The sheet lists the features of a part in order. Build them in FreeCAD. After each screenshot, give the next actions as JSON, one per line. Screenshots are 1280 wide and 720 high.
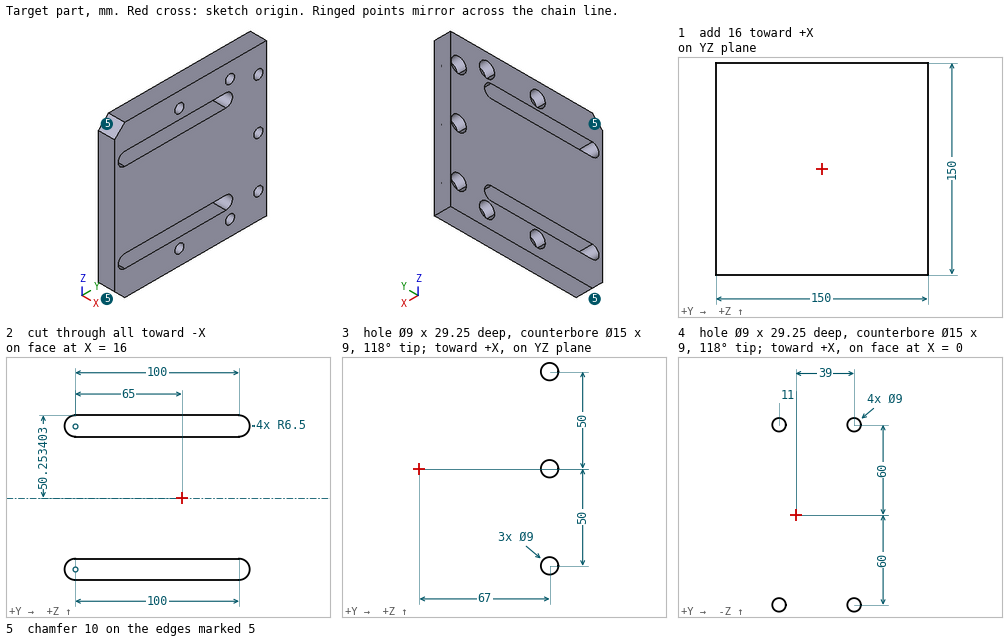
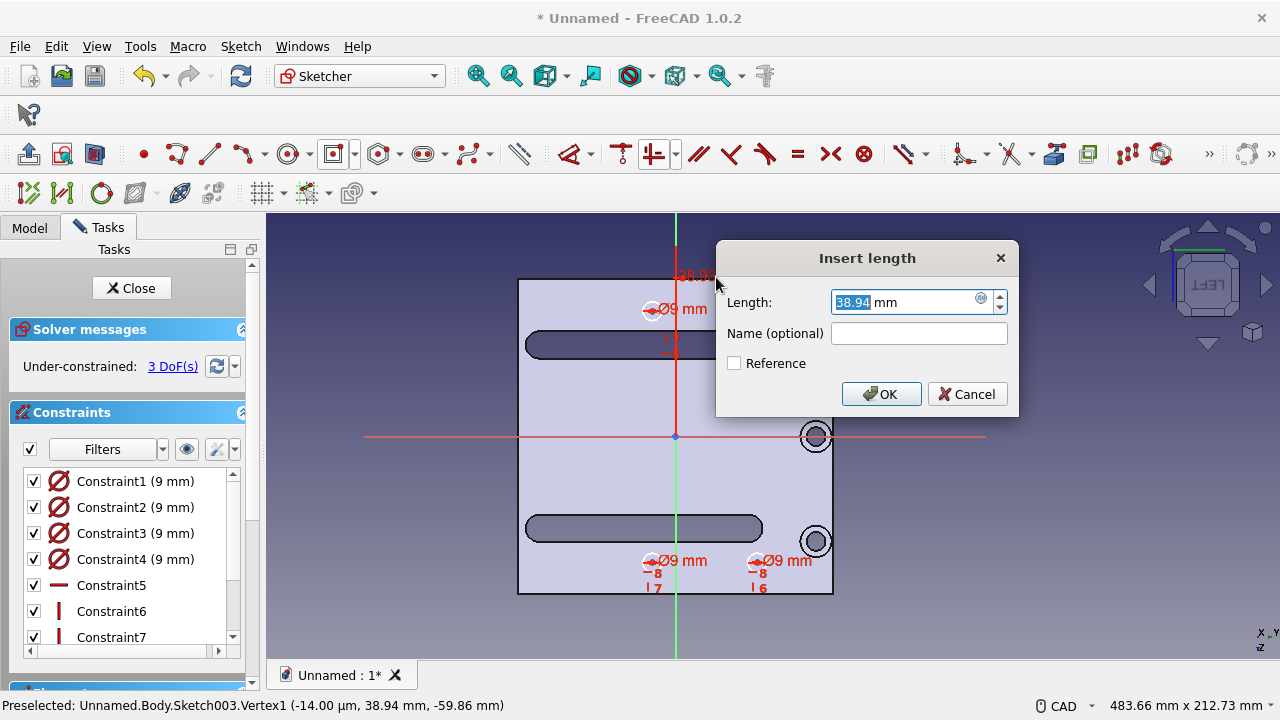
{"action": "type", "text": "39"}
{"action": "key", "text": "Return"}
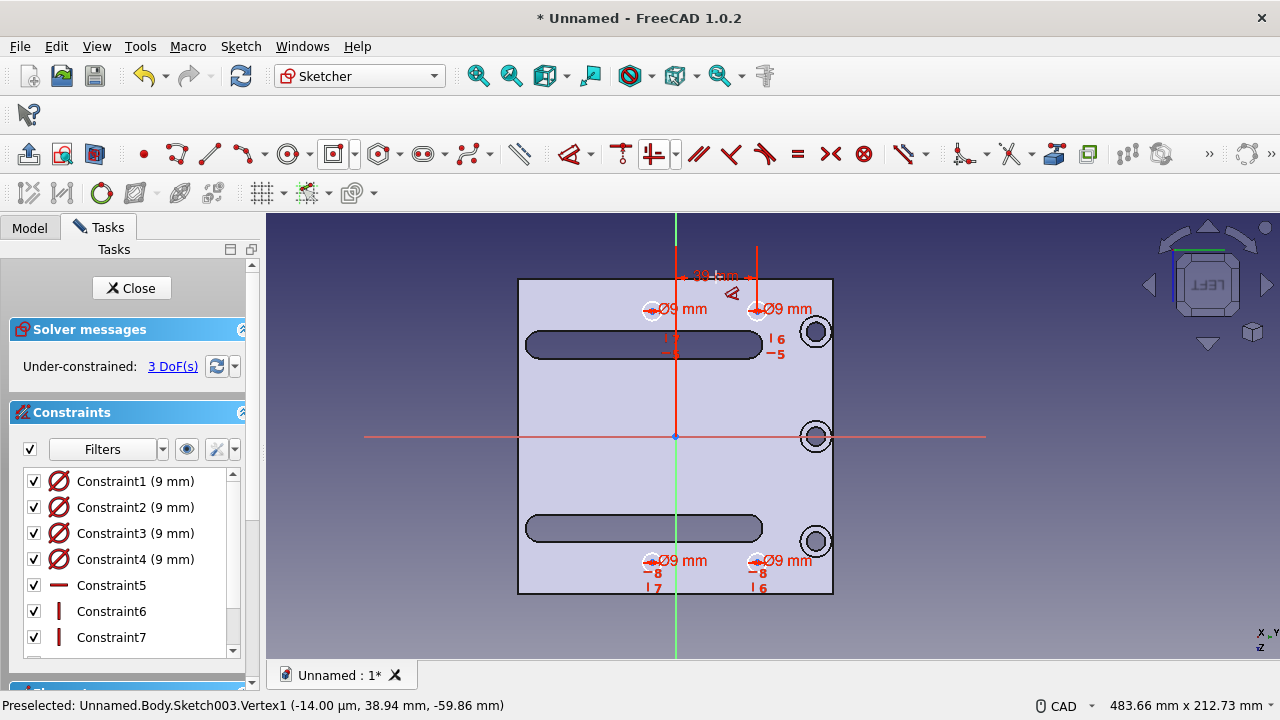
{"action": "left_click", "coordinate": [757, 311]}
{"action": "left_click", "coordinate": [791, 374]}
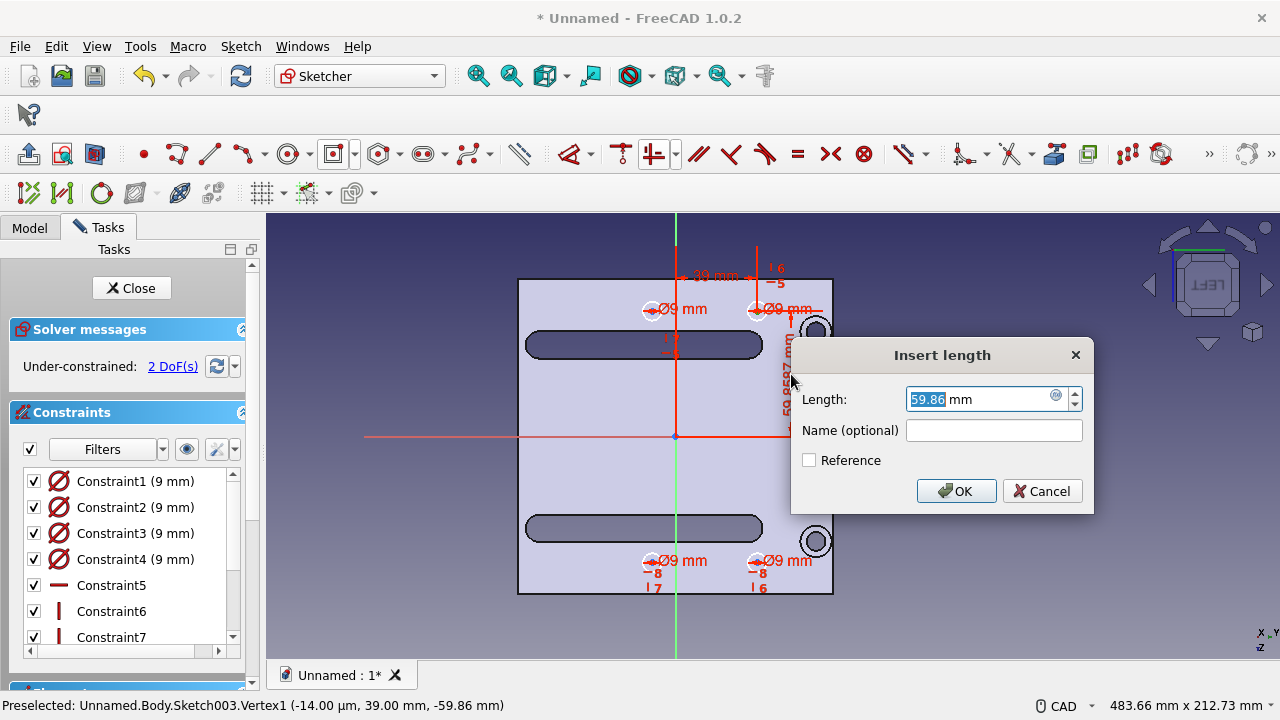
{"action": "type", "text": "60"}
{"action": "key", "text": "Return"}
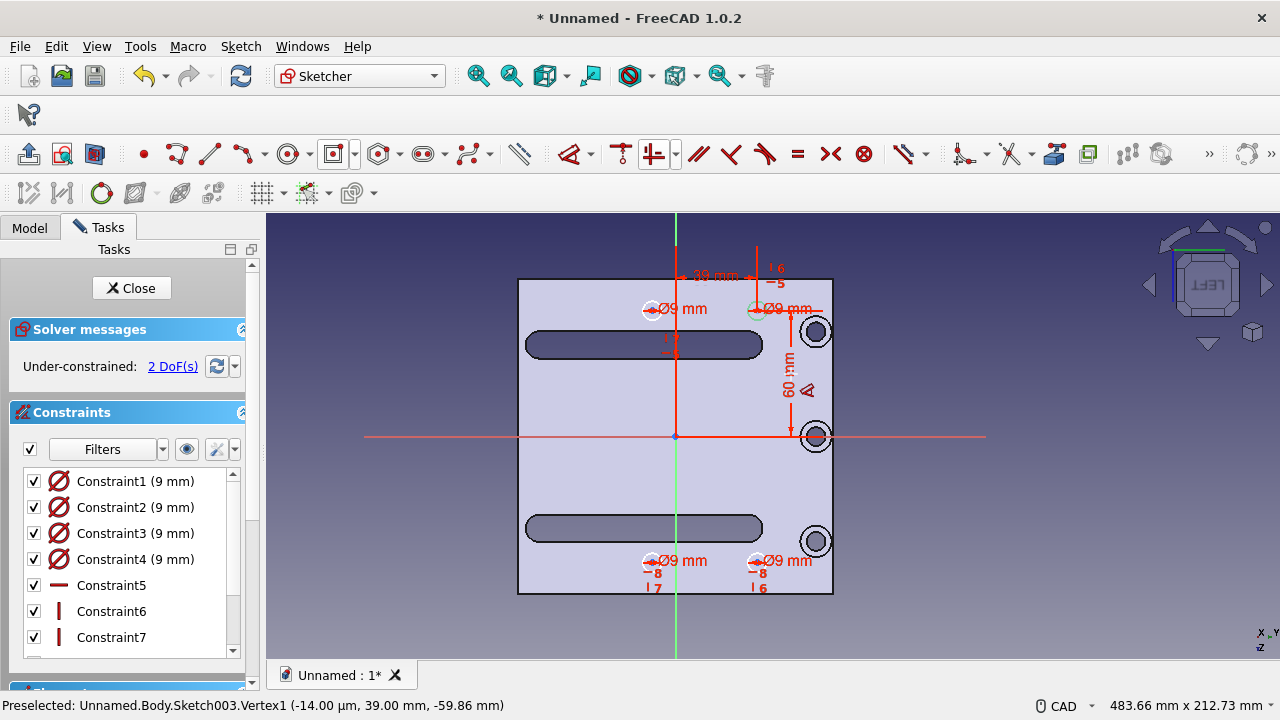
{"action": "scroll", "coordinate": [652, 311], "scroll_direction": "up", "scroll_amount": 3}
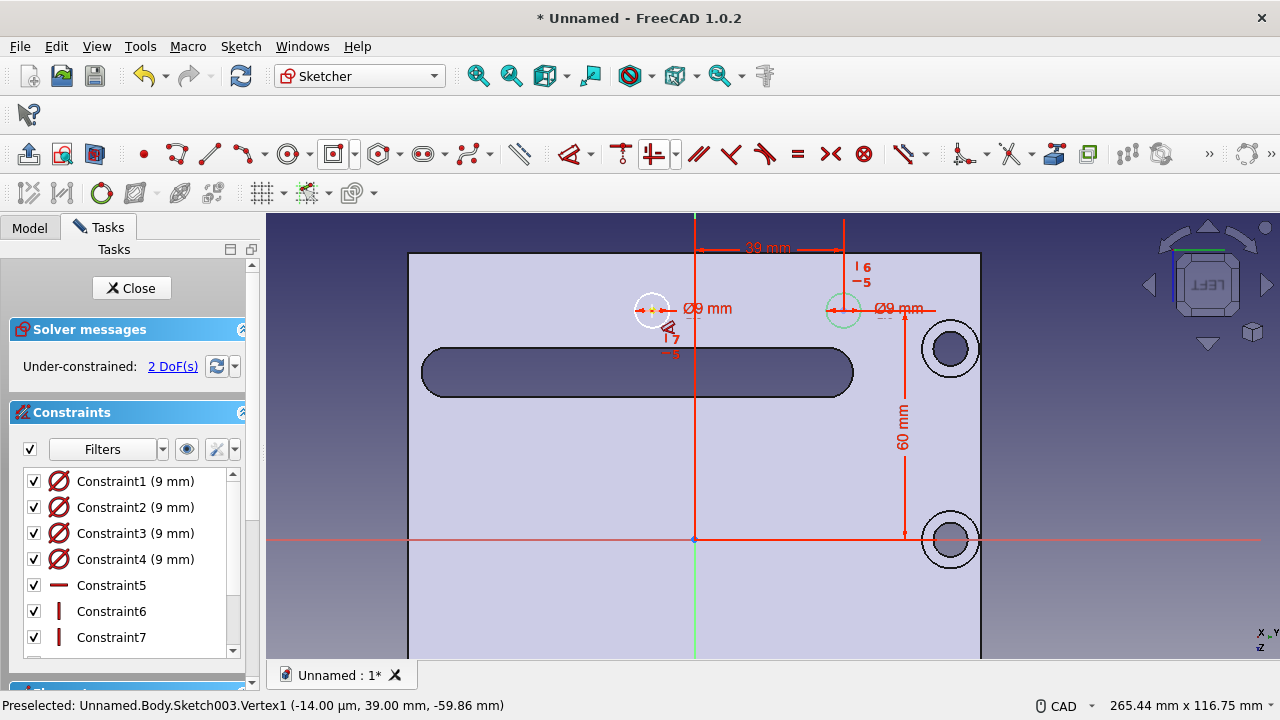
{"action": "left_click", "coordinate": [652, 311]}
{"action": "left_click", "coordinate": [673, 277]}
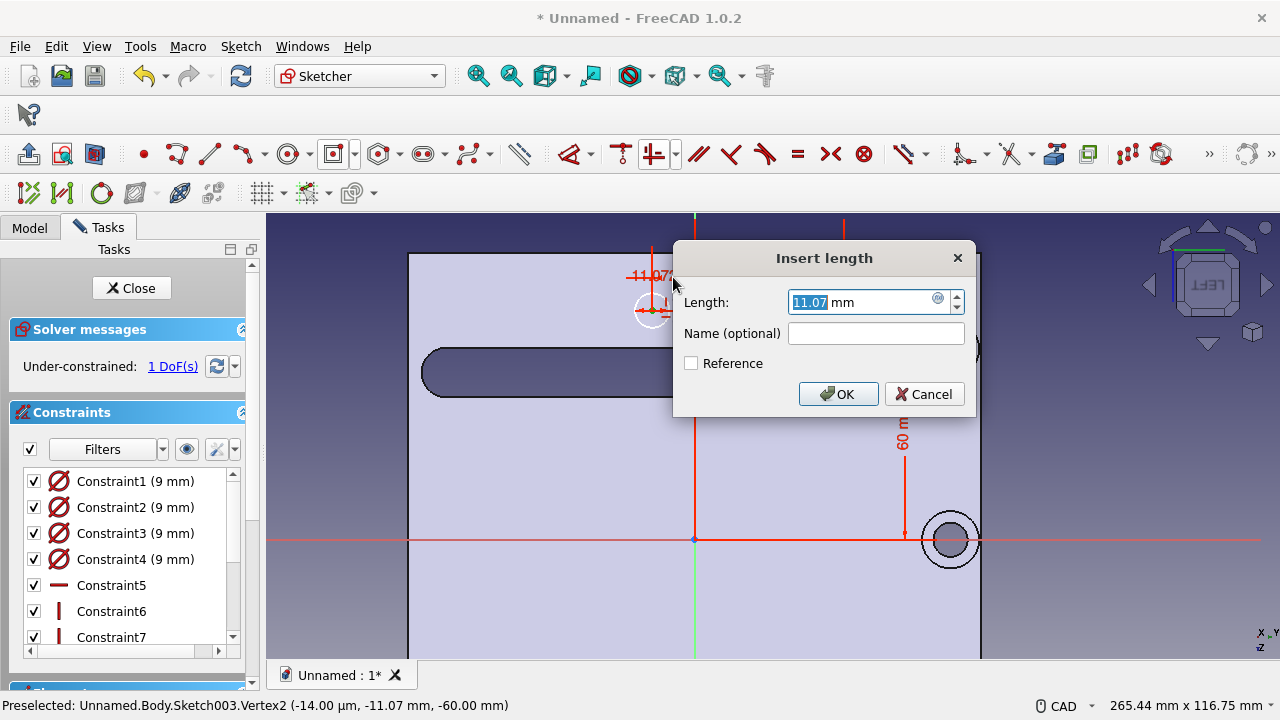
{"action": "type", "text": "11"}
{"action": "key", "text": "Return"}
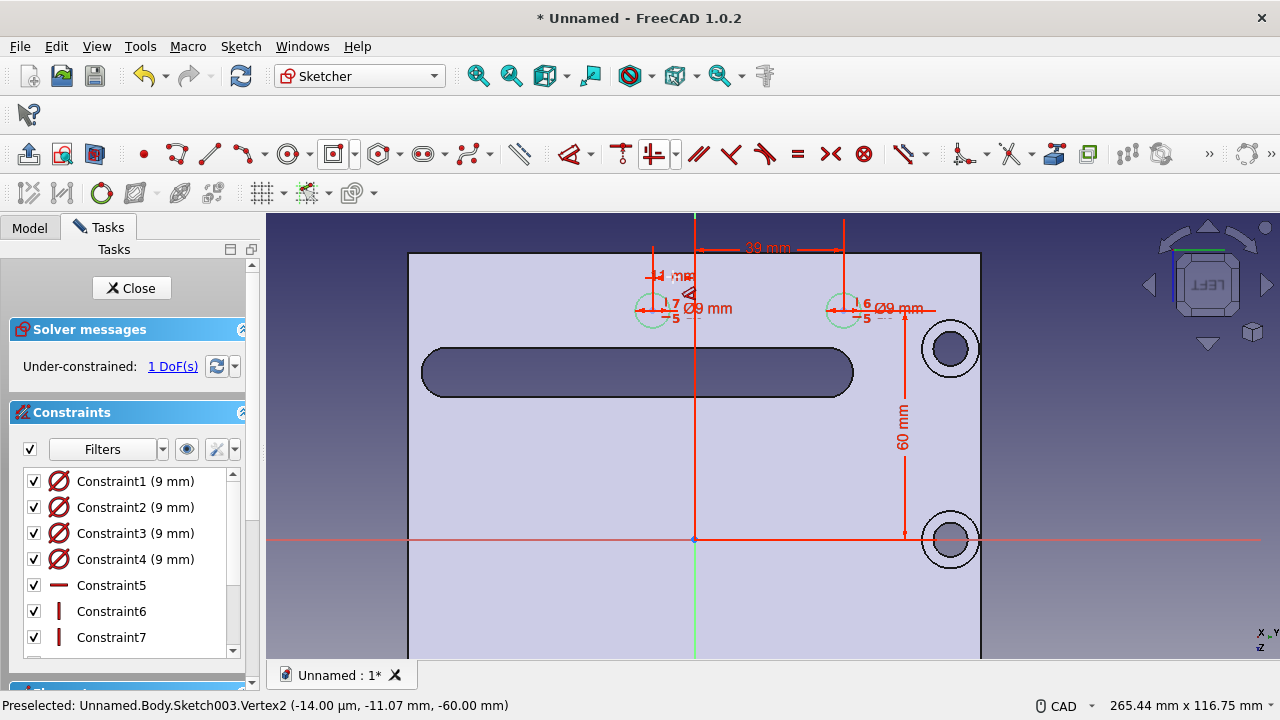
{"action": "scroll", "coordinate": [651, 310], "scroll_direction": "down", "scroll_amount": 3}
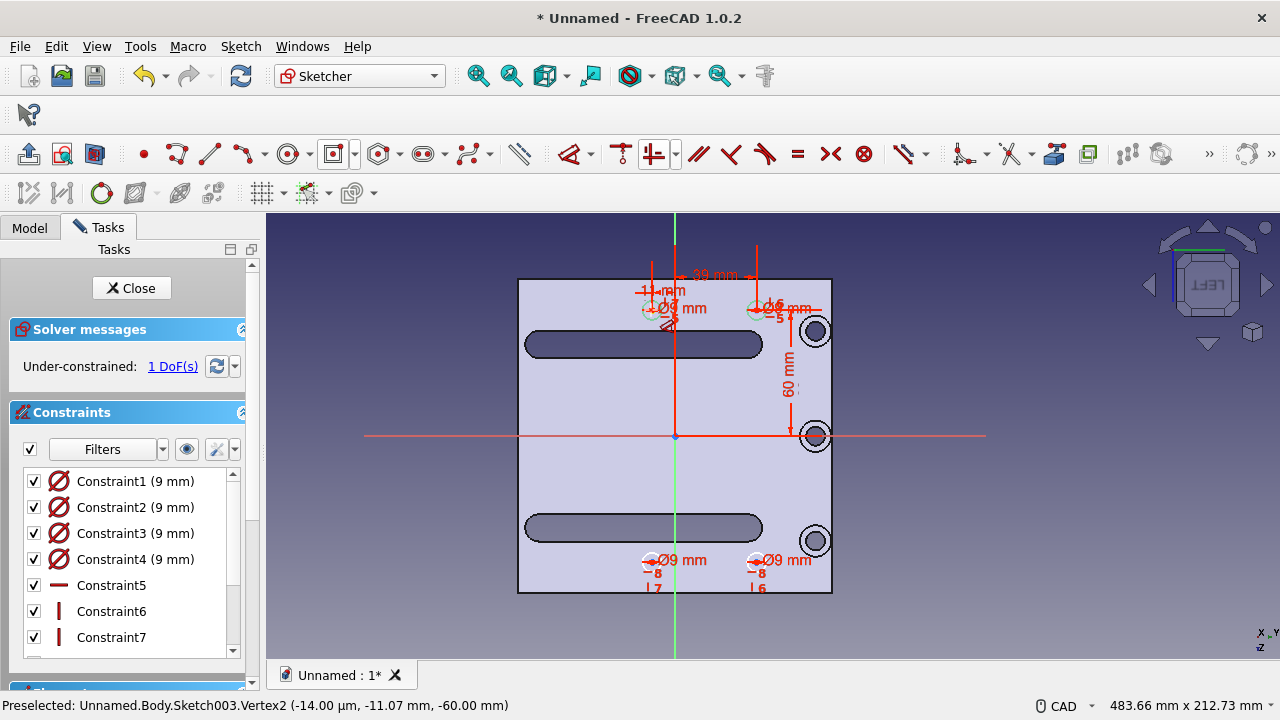
{"action": "left_click", "coordinate": [757, 562]}
{"action": "left_click", "coordinate": [791, 499]}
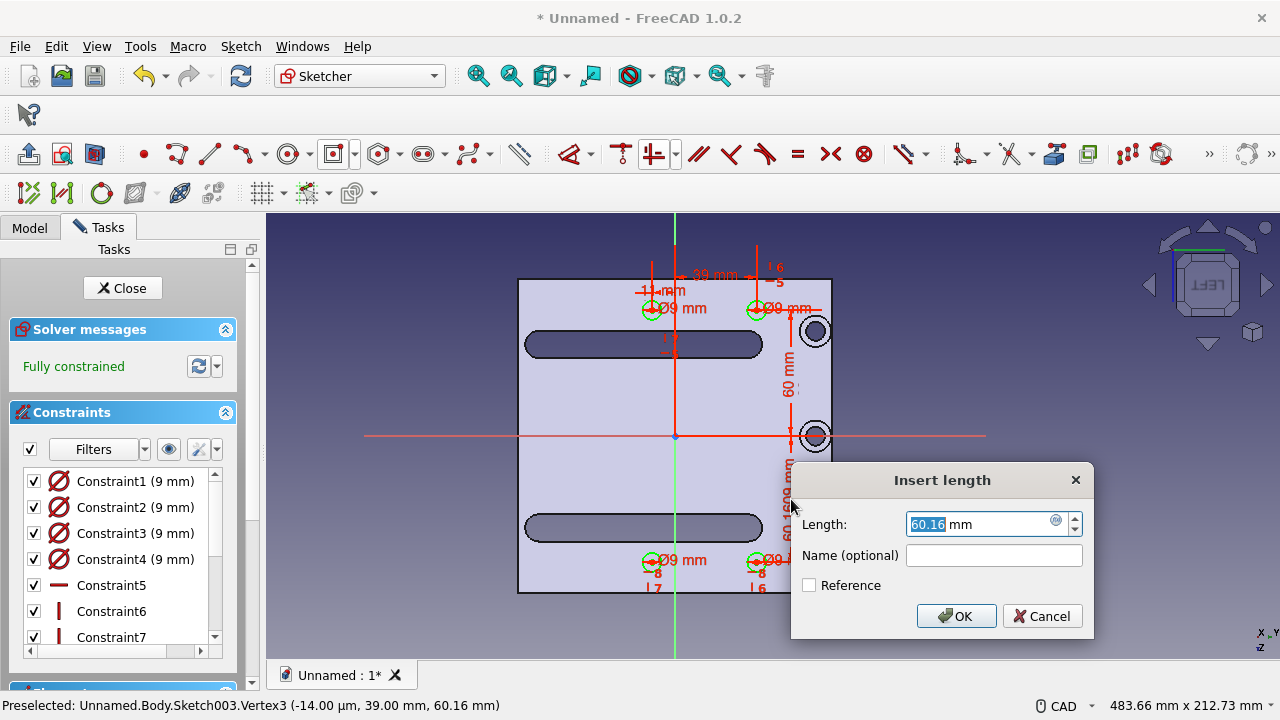
{"action": "type", "text": "60"}
{"action": "key", "text": "Return"}
{"action": "key", "text": "Escape"}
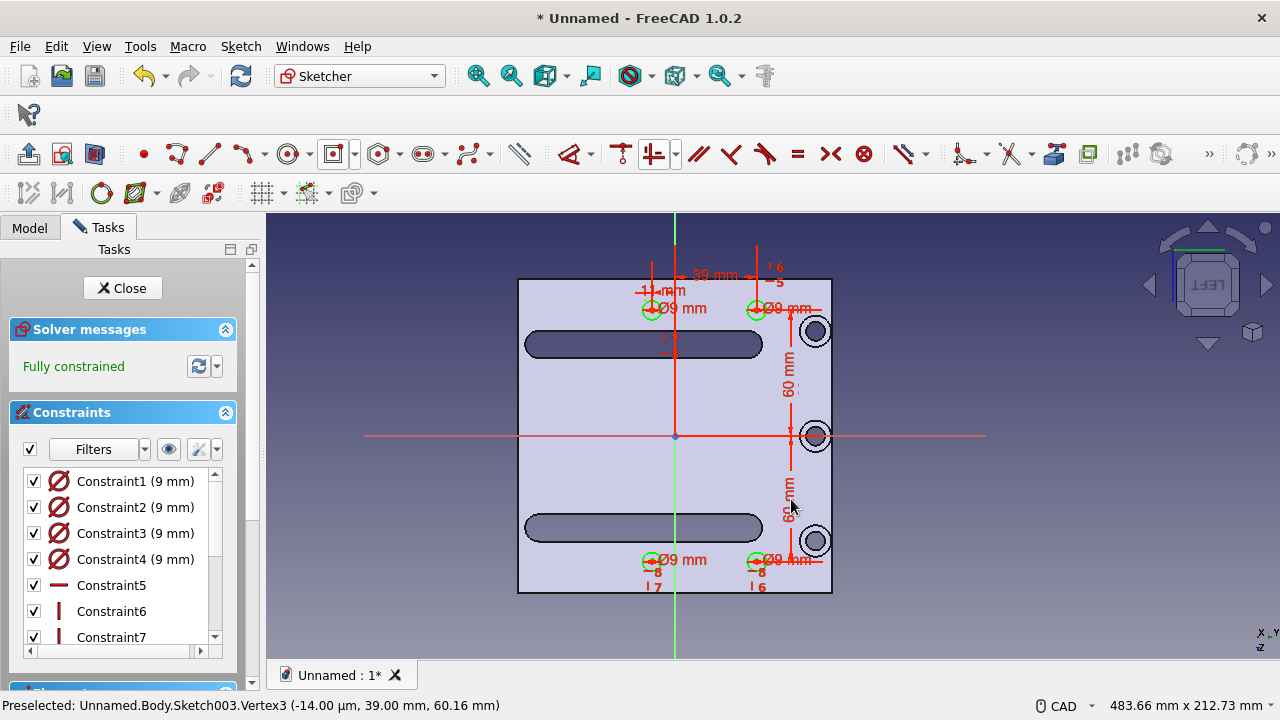
{"action": "left_click", "coordinate": [123, 288]}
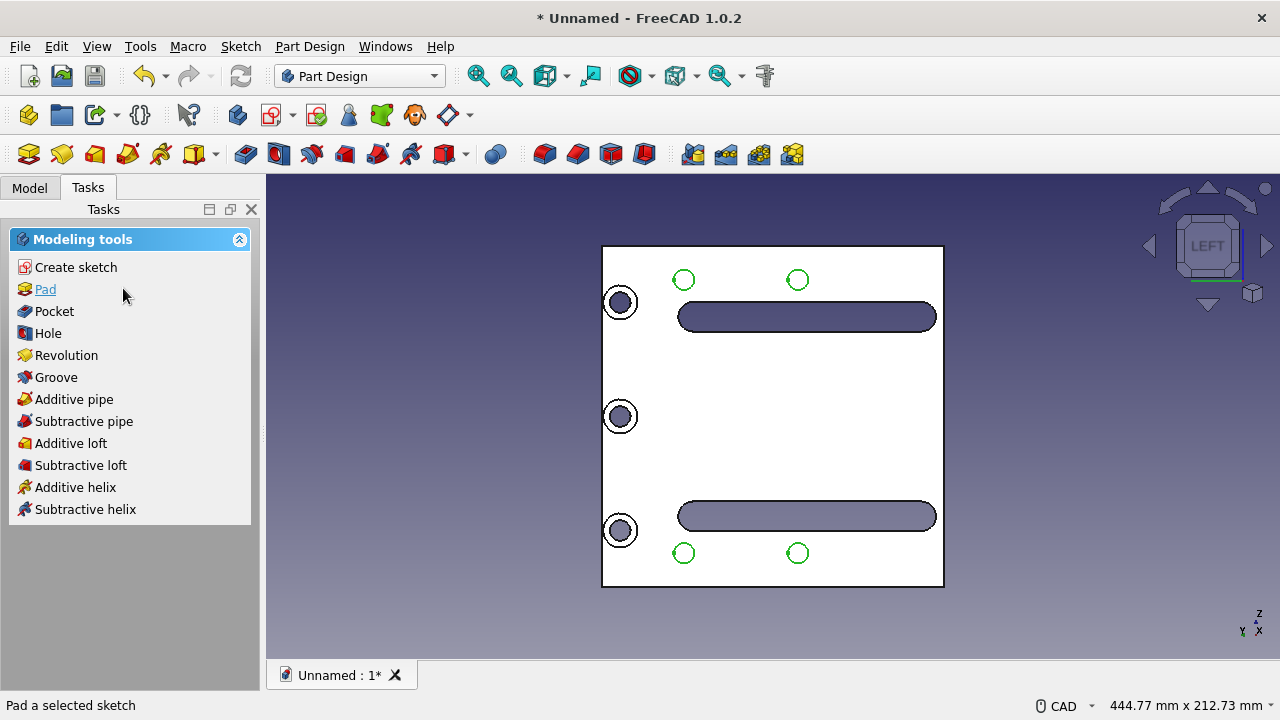
{"action": "left_click", "coordinate": [279, 154]}